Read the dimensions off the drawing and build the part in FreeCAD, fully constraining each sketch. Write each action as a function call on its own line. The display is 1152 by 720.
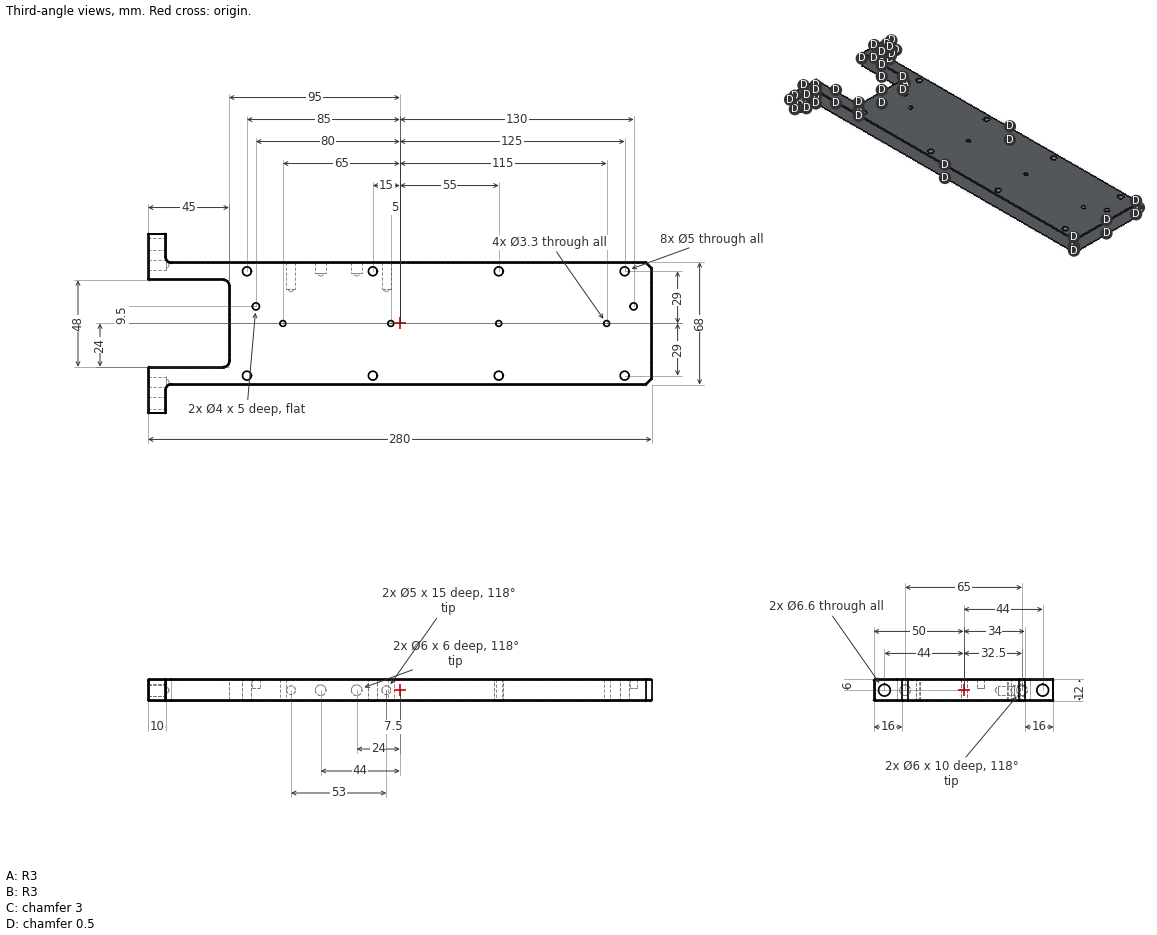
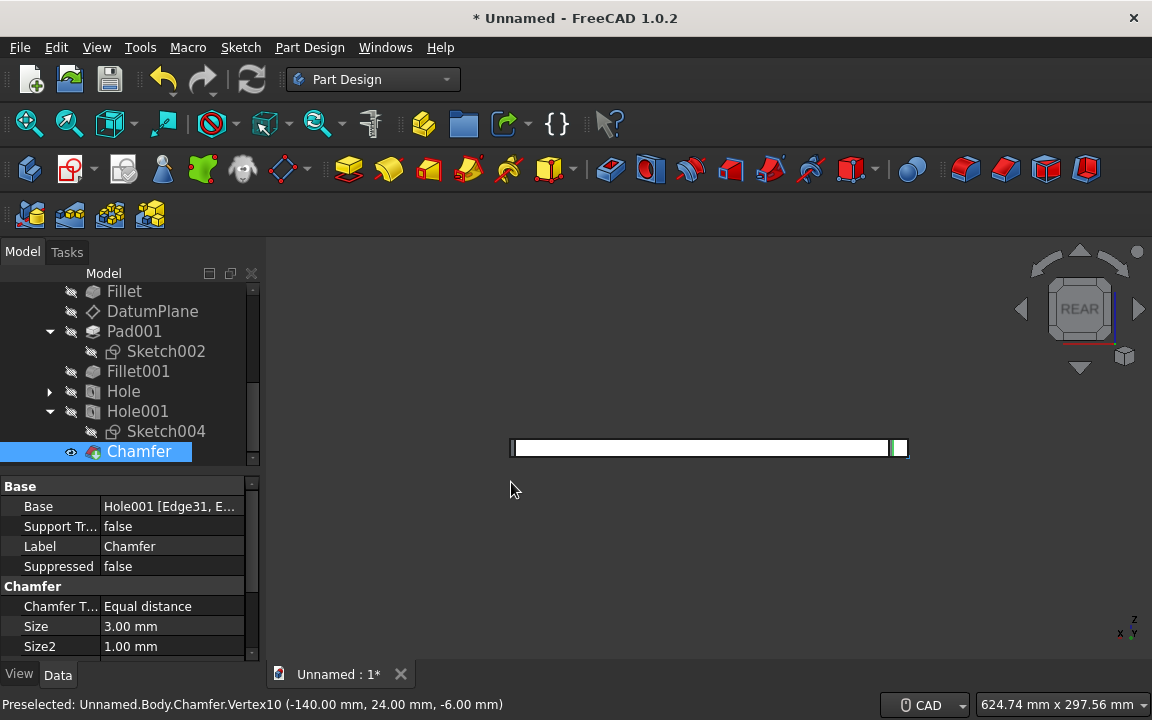
key(v)
key(f)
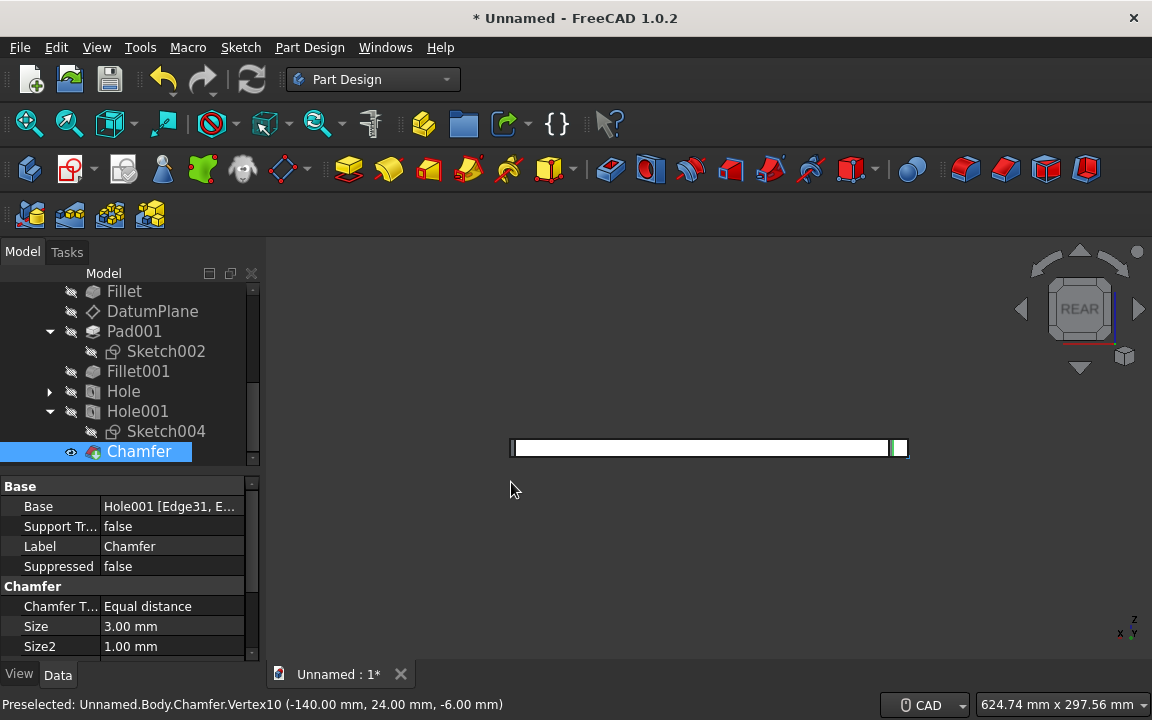
click(908, 447, ctrl)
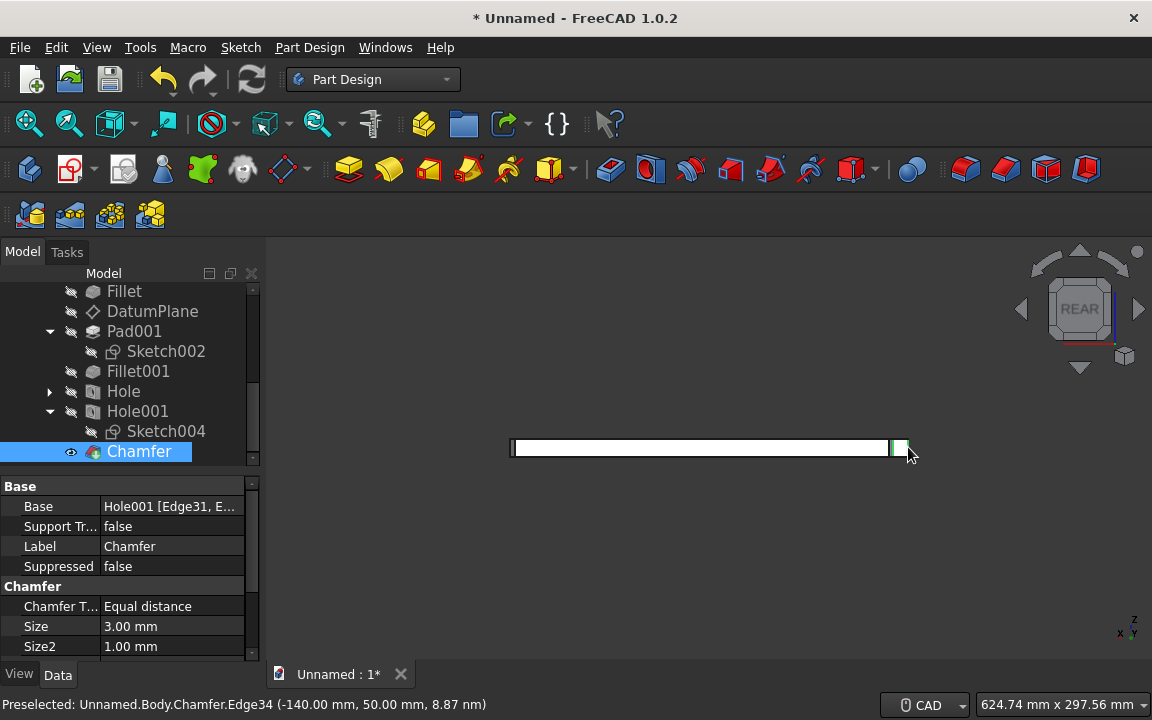
scroll(908, 447, up, 5)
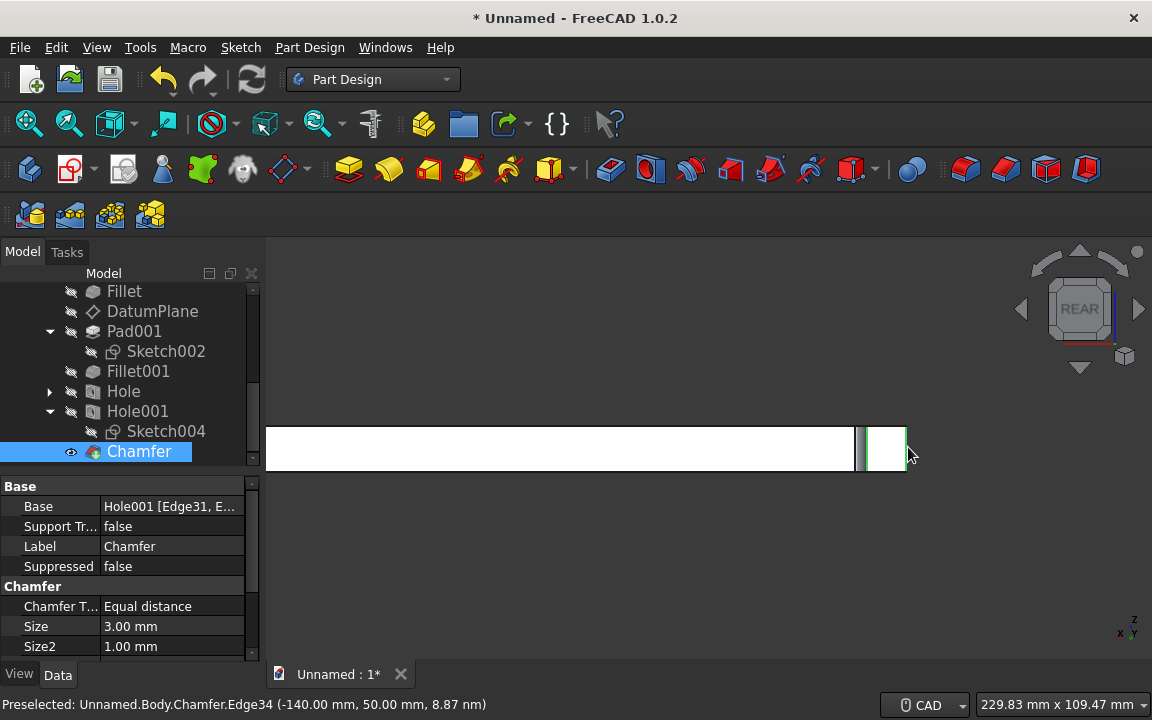
key(v)
key(f)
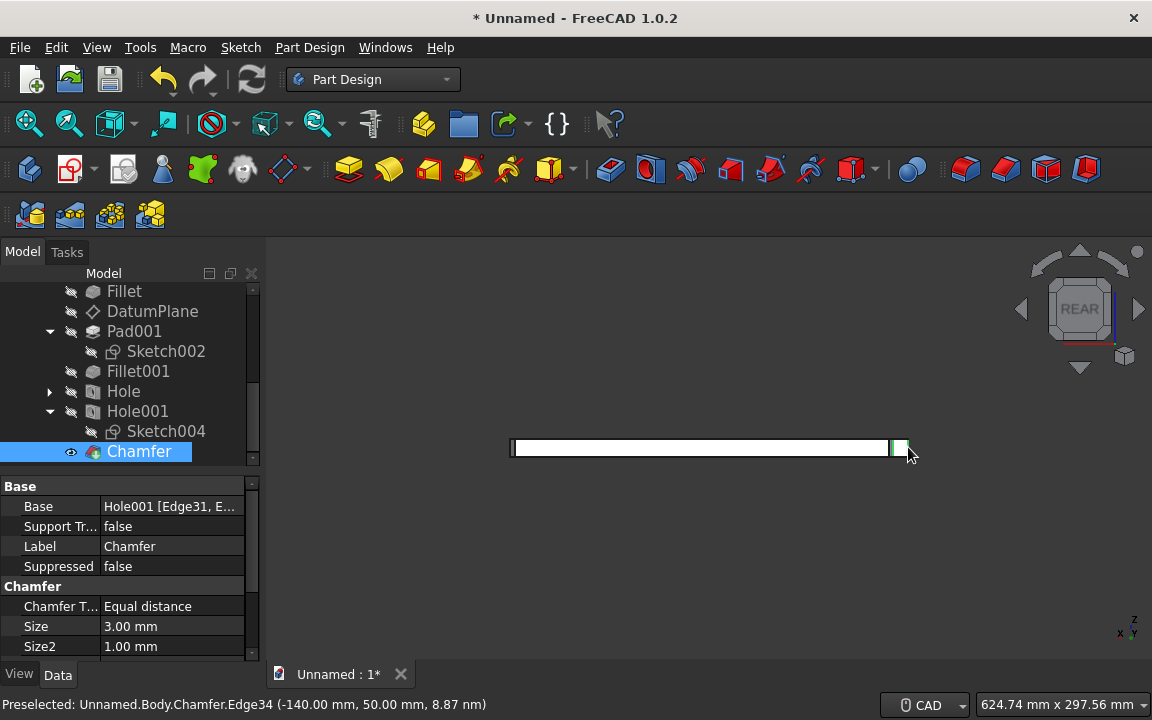
key(6)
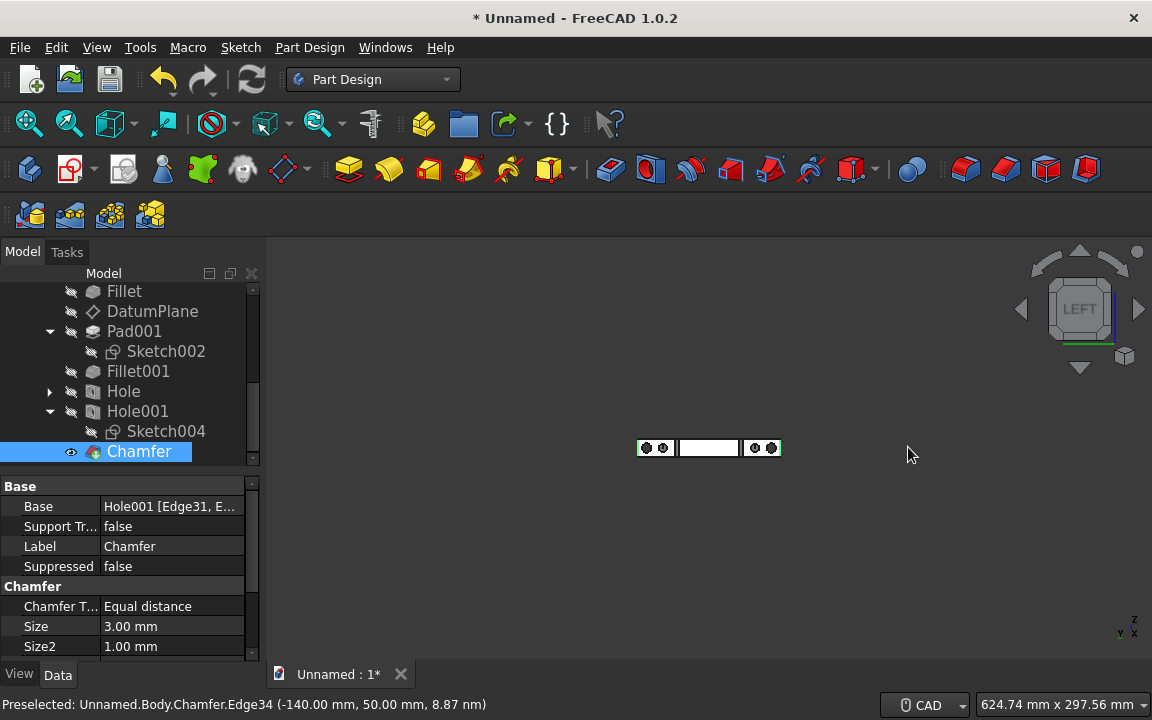
key(v)
key(f)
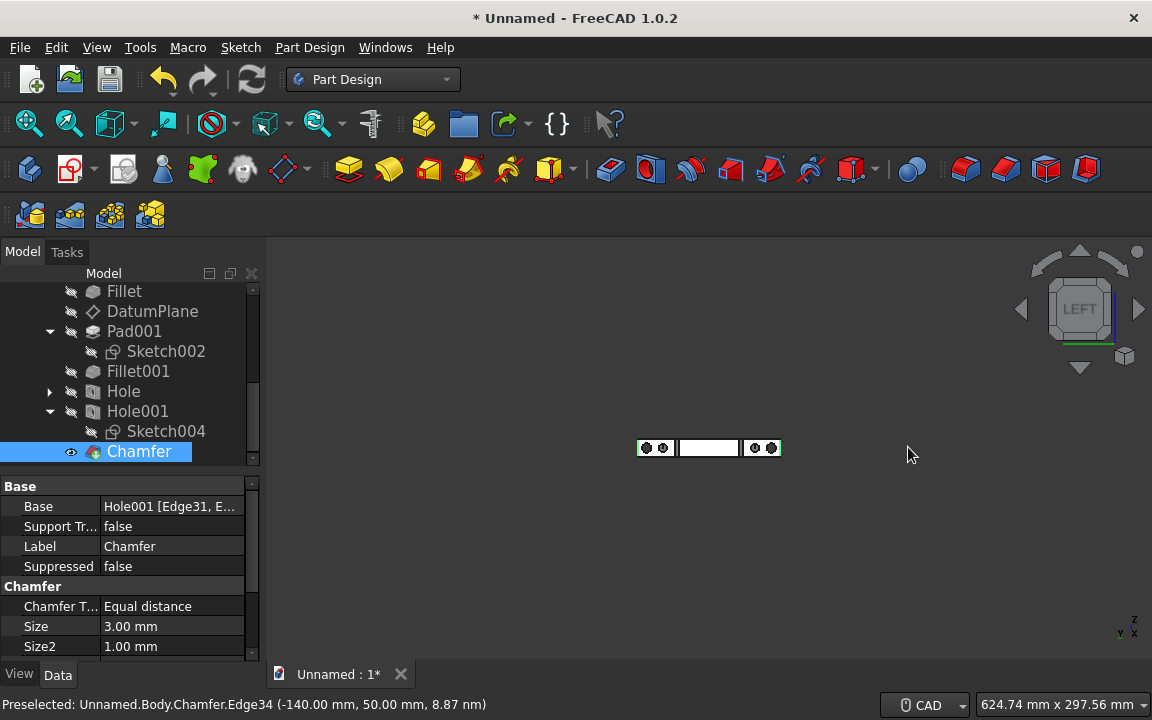
click(675, 447, ctrl)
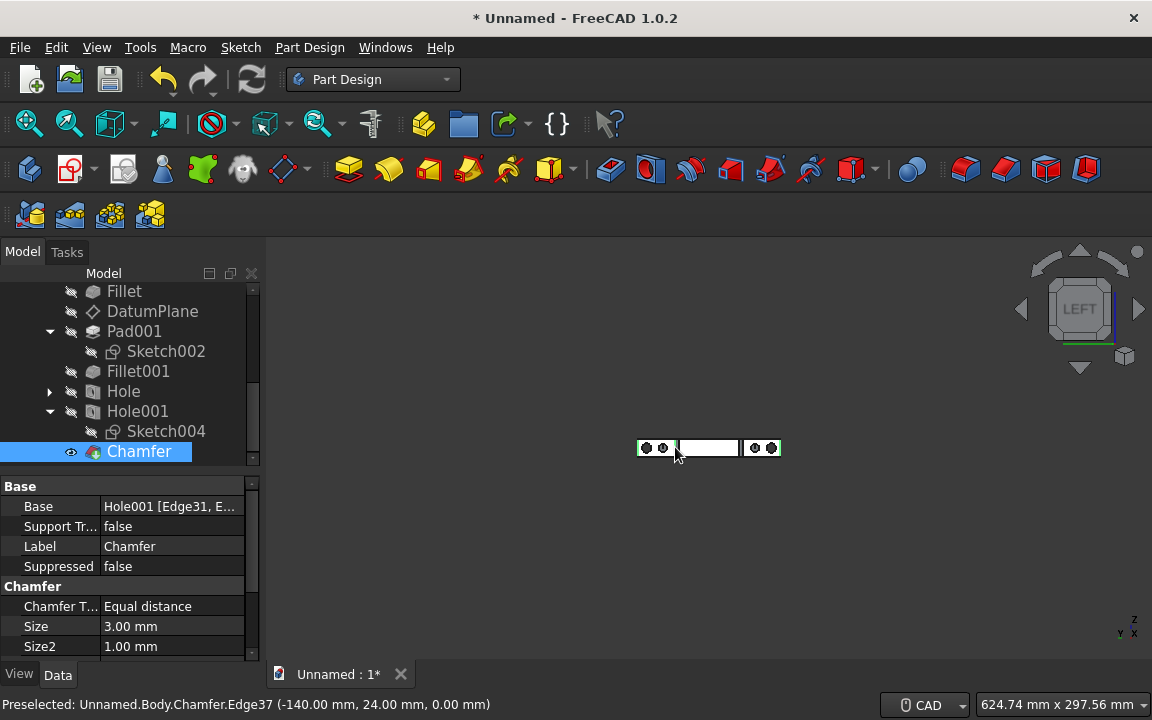
click(743, 447, ctrl)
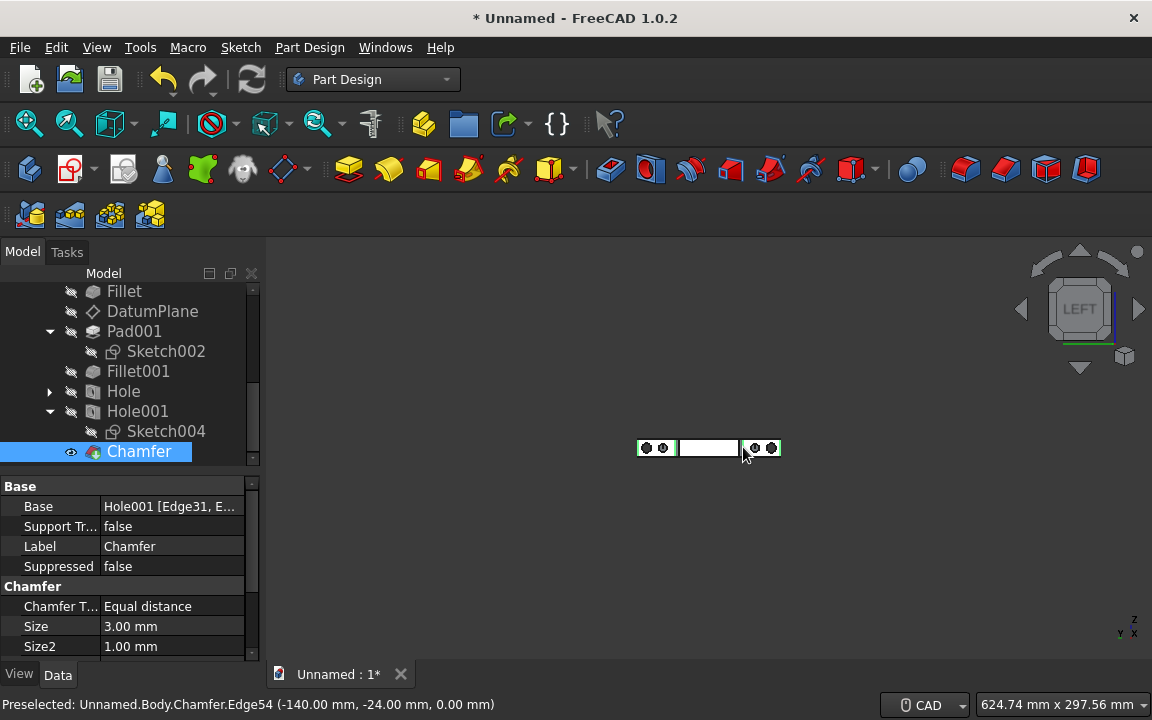
click(1006, 170)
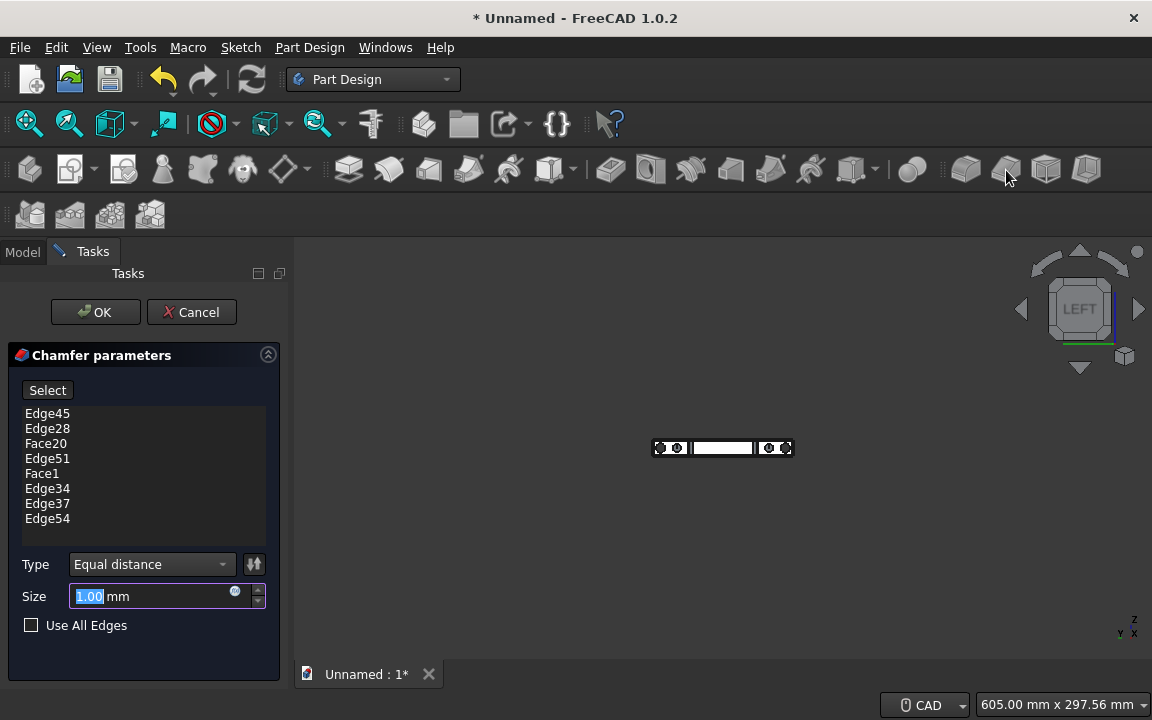
text(0.5)
key(Tab)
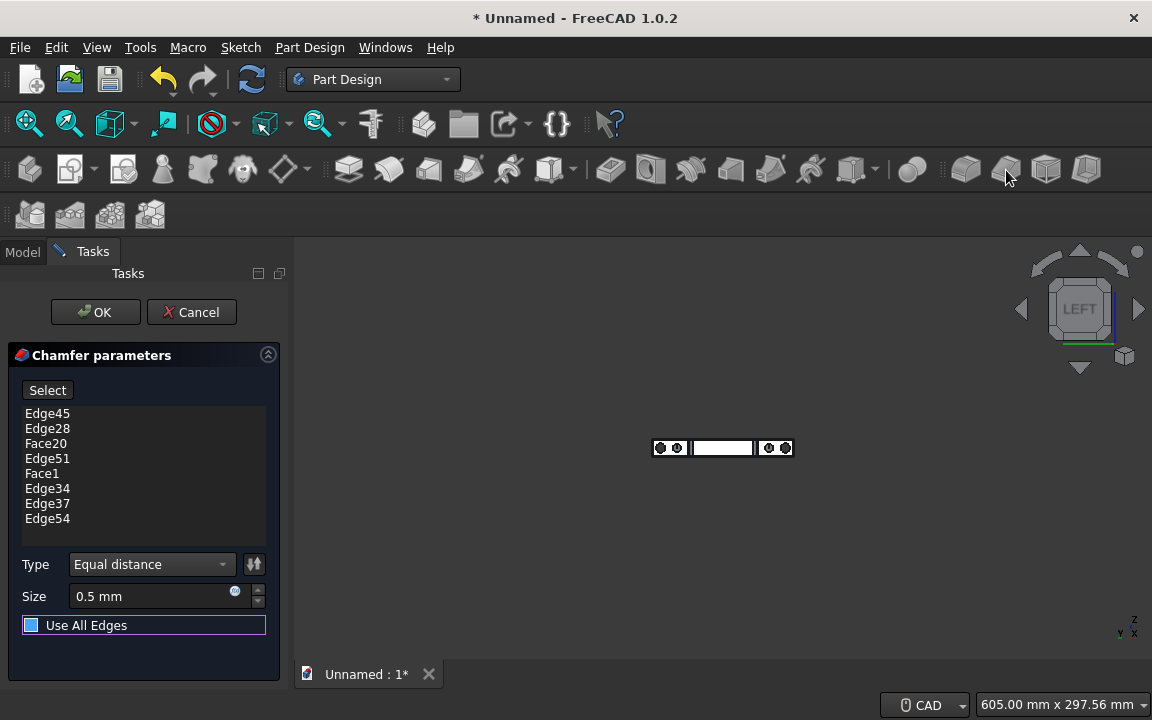
click(96, 312)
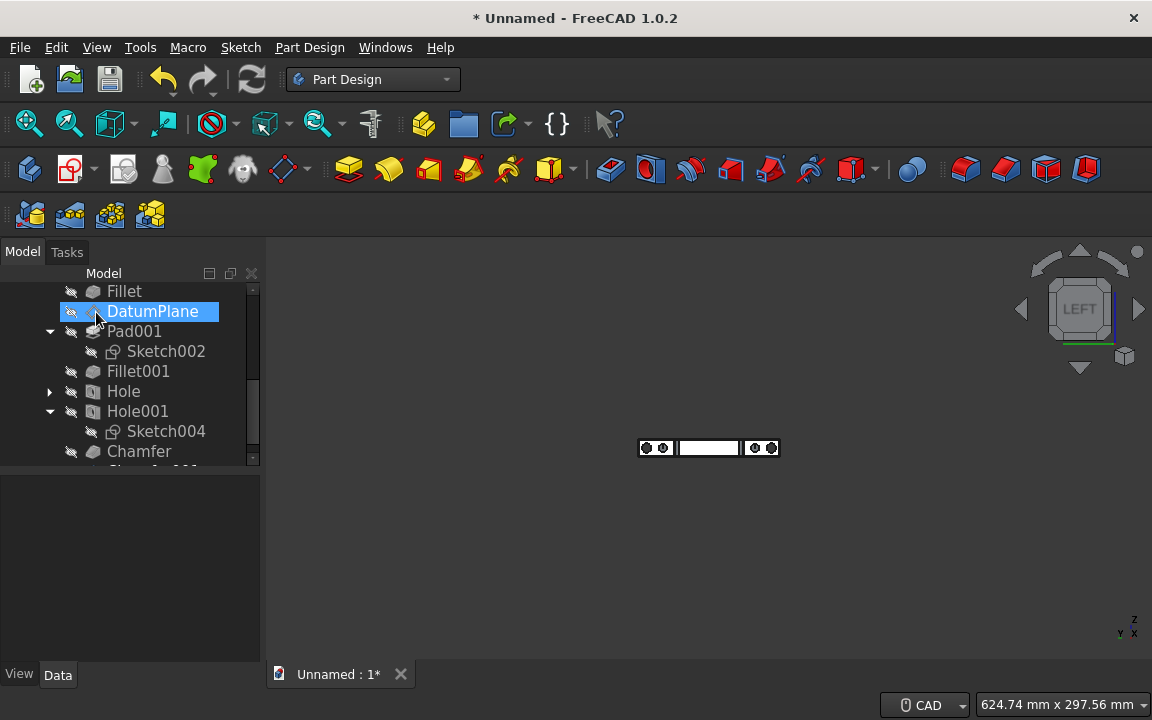
key(v)
key(f)